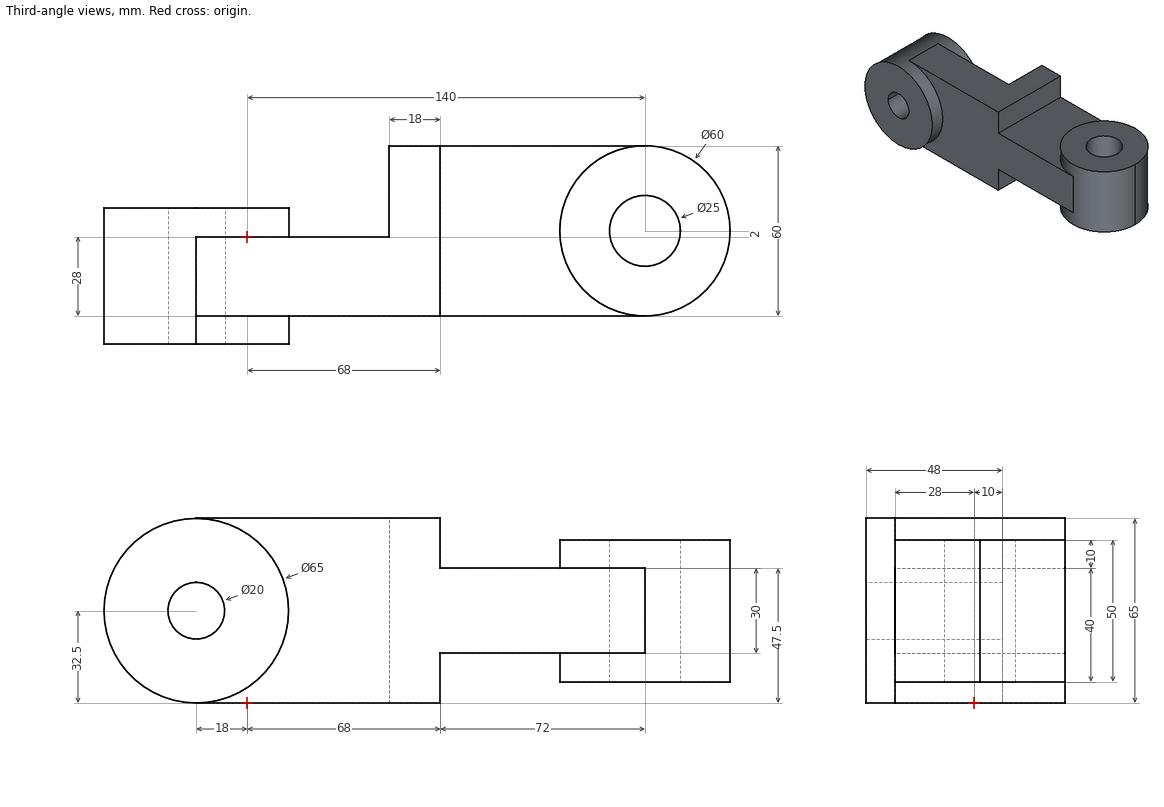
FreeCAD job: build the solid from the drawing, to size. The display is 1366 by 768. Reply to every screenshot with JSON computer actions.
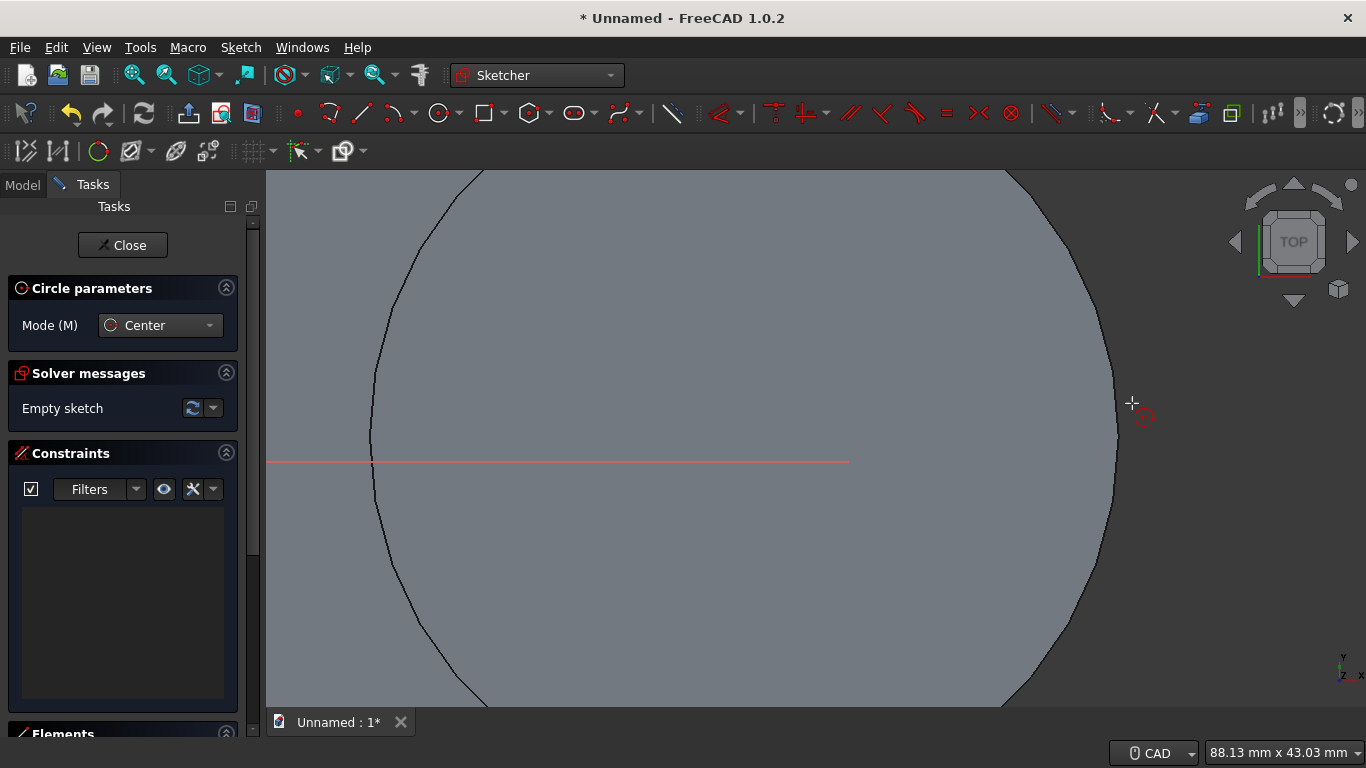
{"action": "left_click", "coordinate": [744, 437]}
{"action": "left_click", "coordinate": [855, 326]}
{"action": "key", "text": "Escape"}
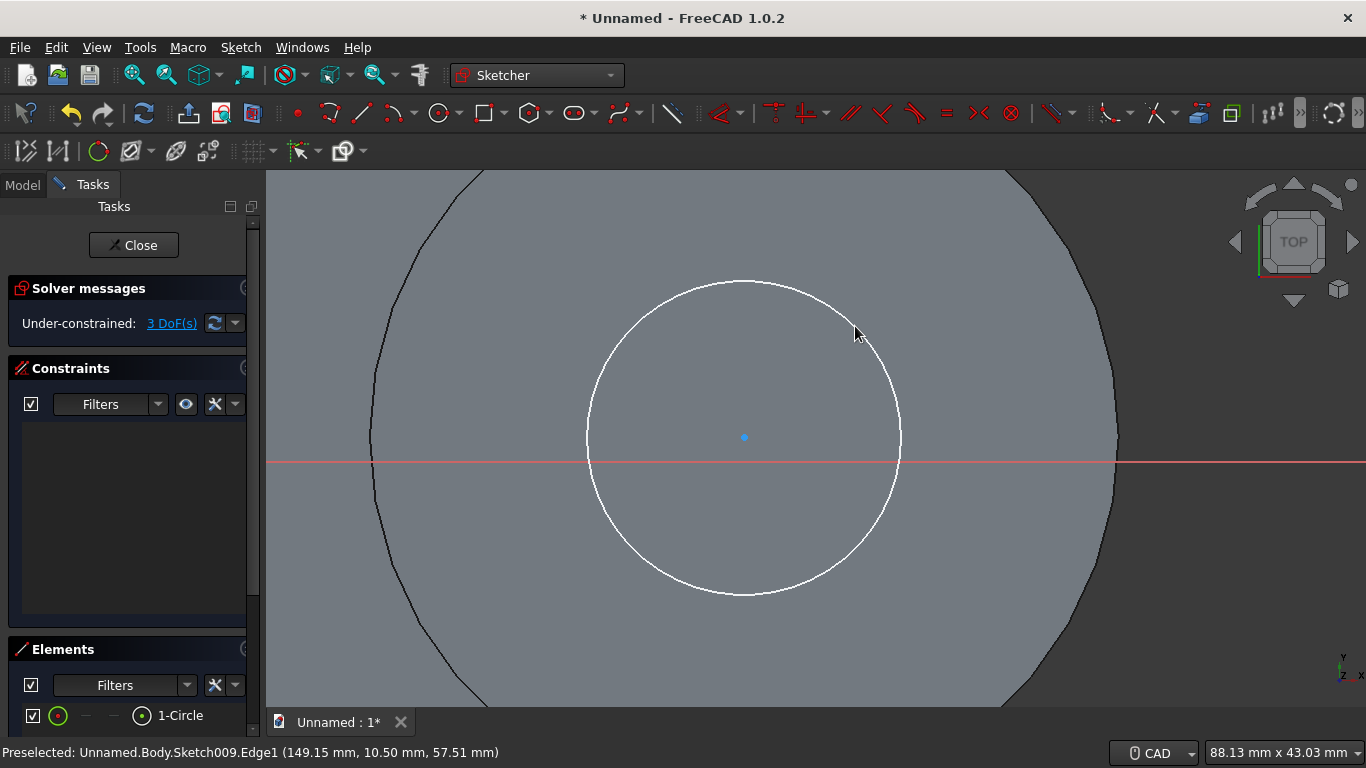
{"action": "key", "text": "d"}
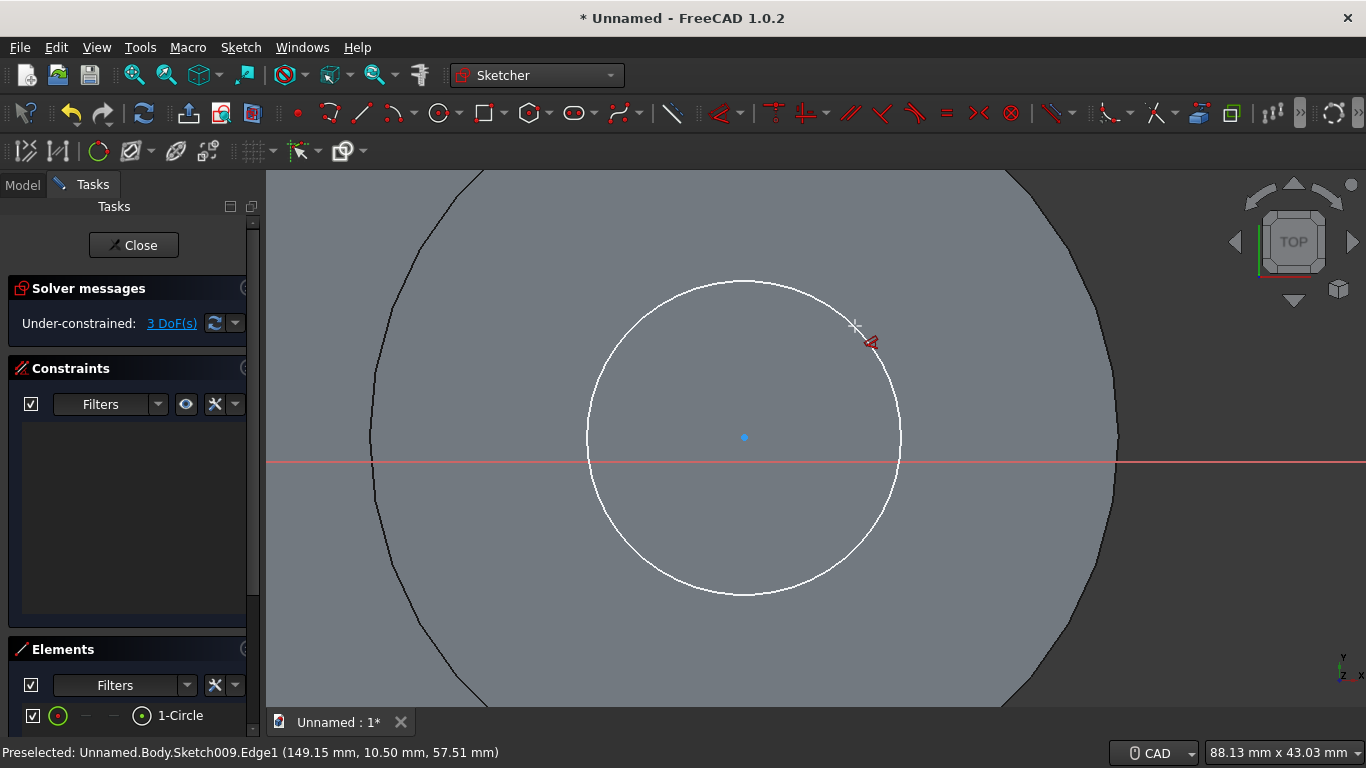
{"action": "left_click", "coordinate": [855, 327]}
{"action": "left_click", "coordinate": [878, 304]}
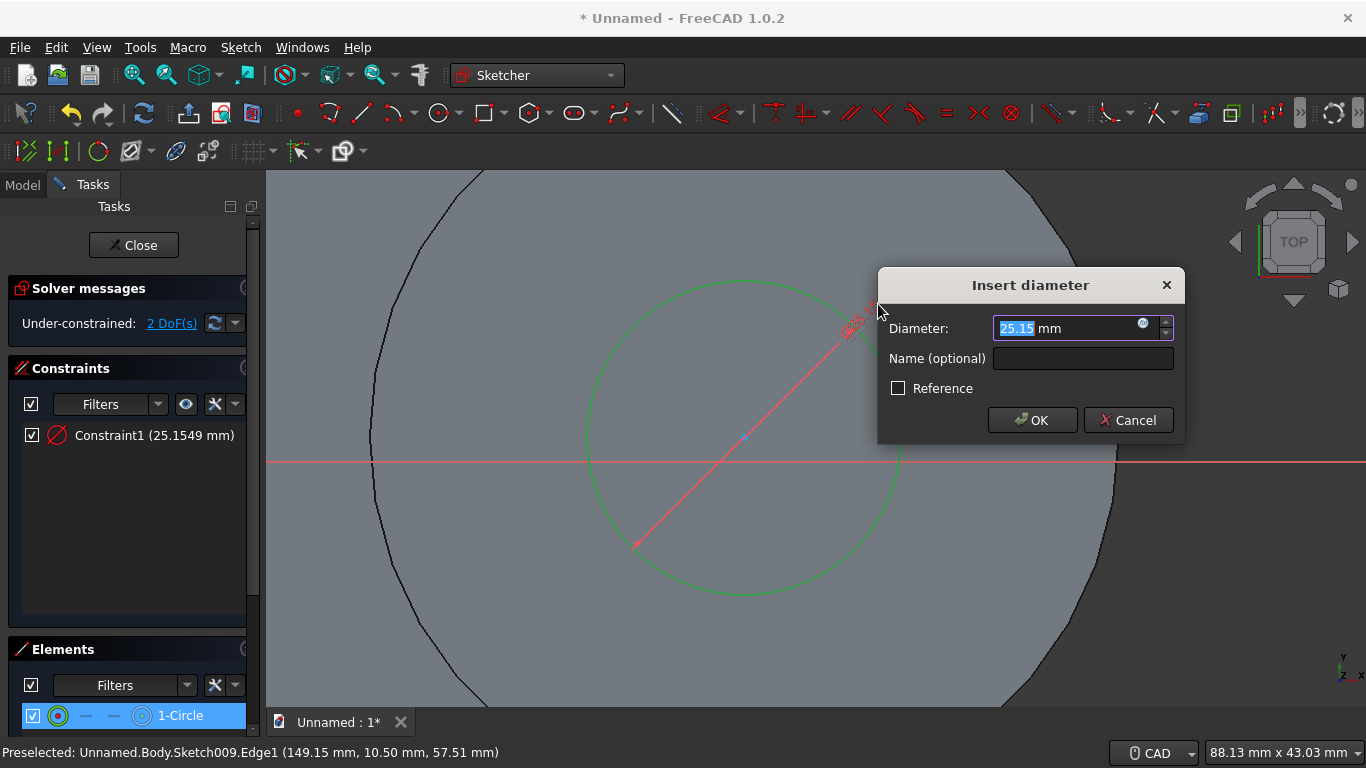
{"action": "type", "text": "25"}
{"action": "key", "text": "Return"}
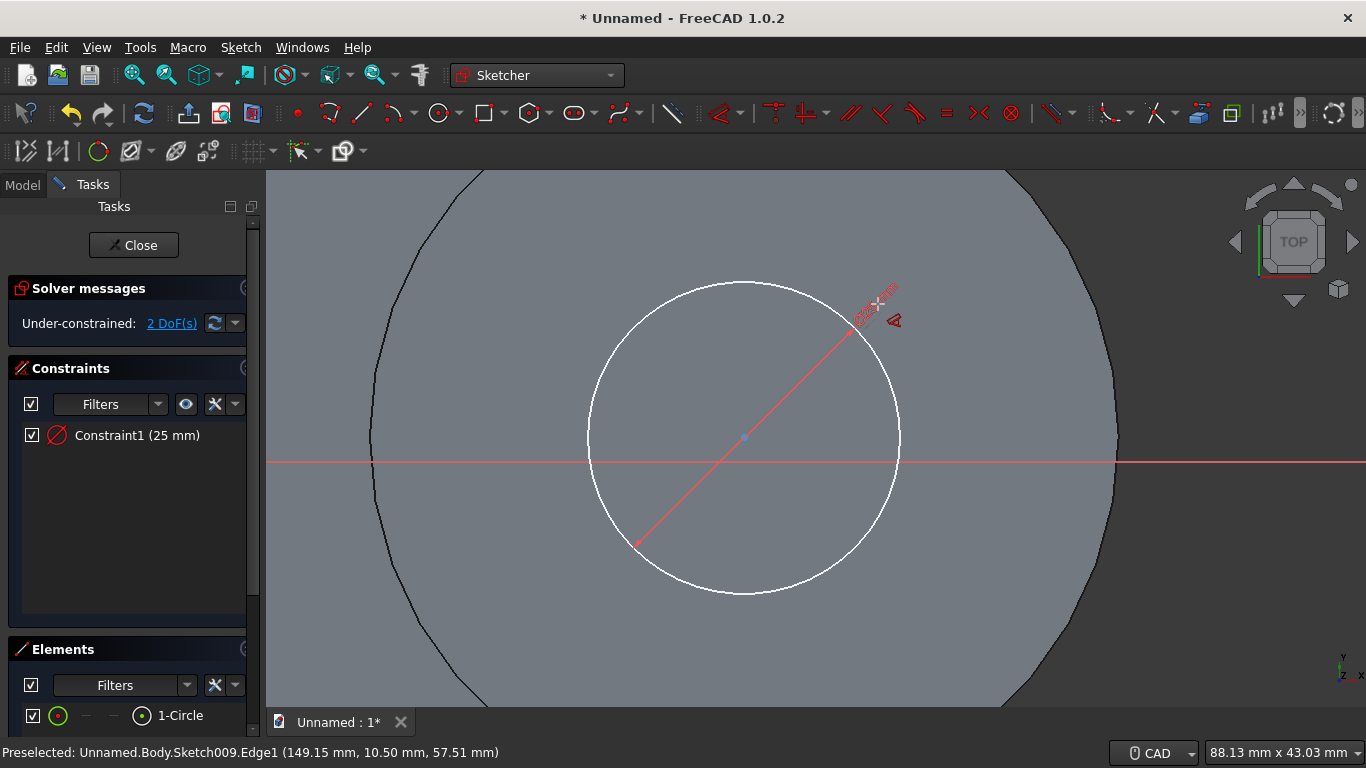
{"action": "scroll", "coordinate": [744, 438], "scroll_direction": "up", "scroll_amount": 3}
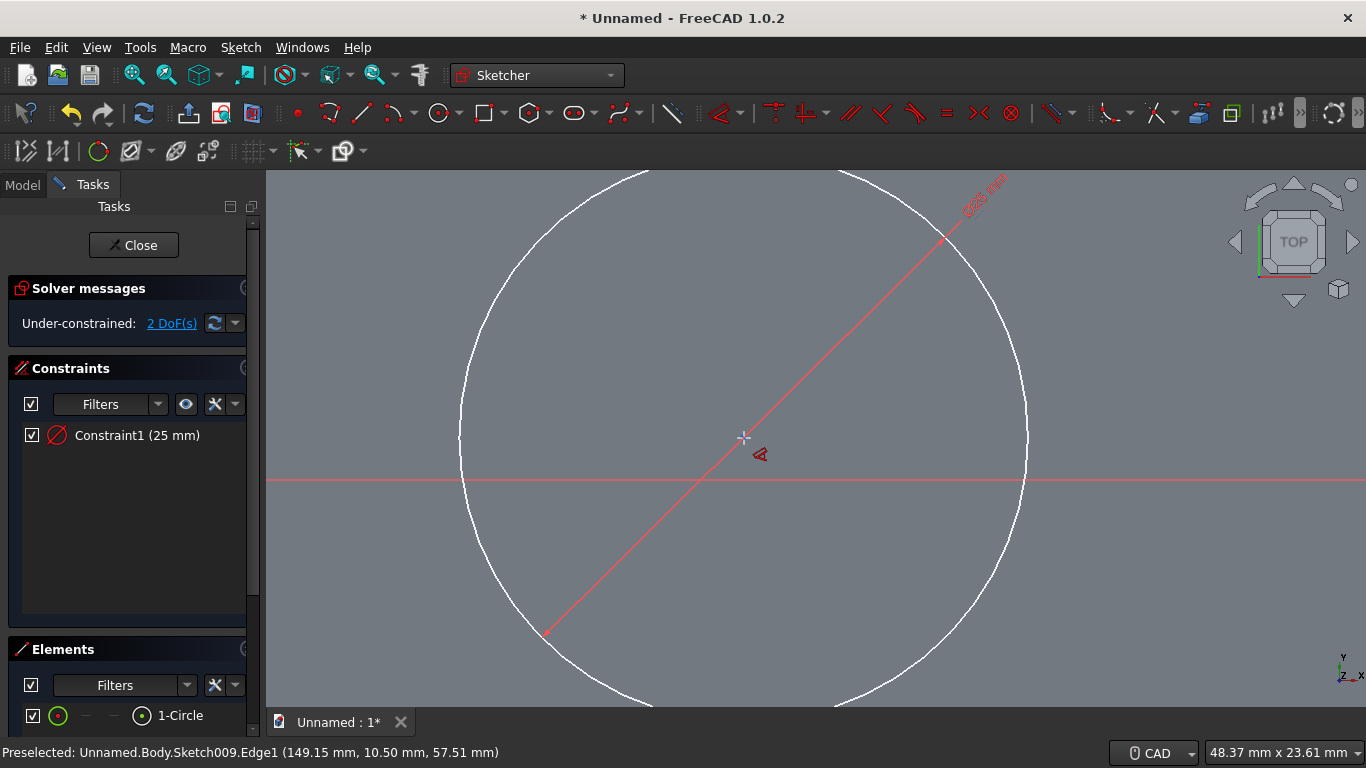
{"action": "left_click", "coordinate": [744, 438]}
{"action": "left_click", "coordinate": [778, 459]}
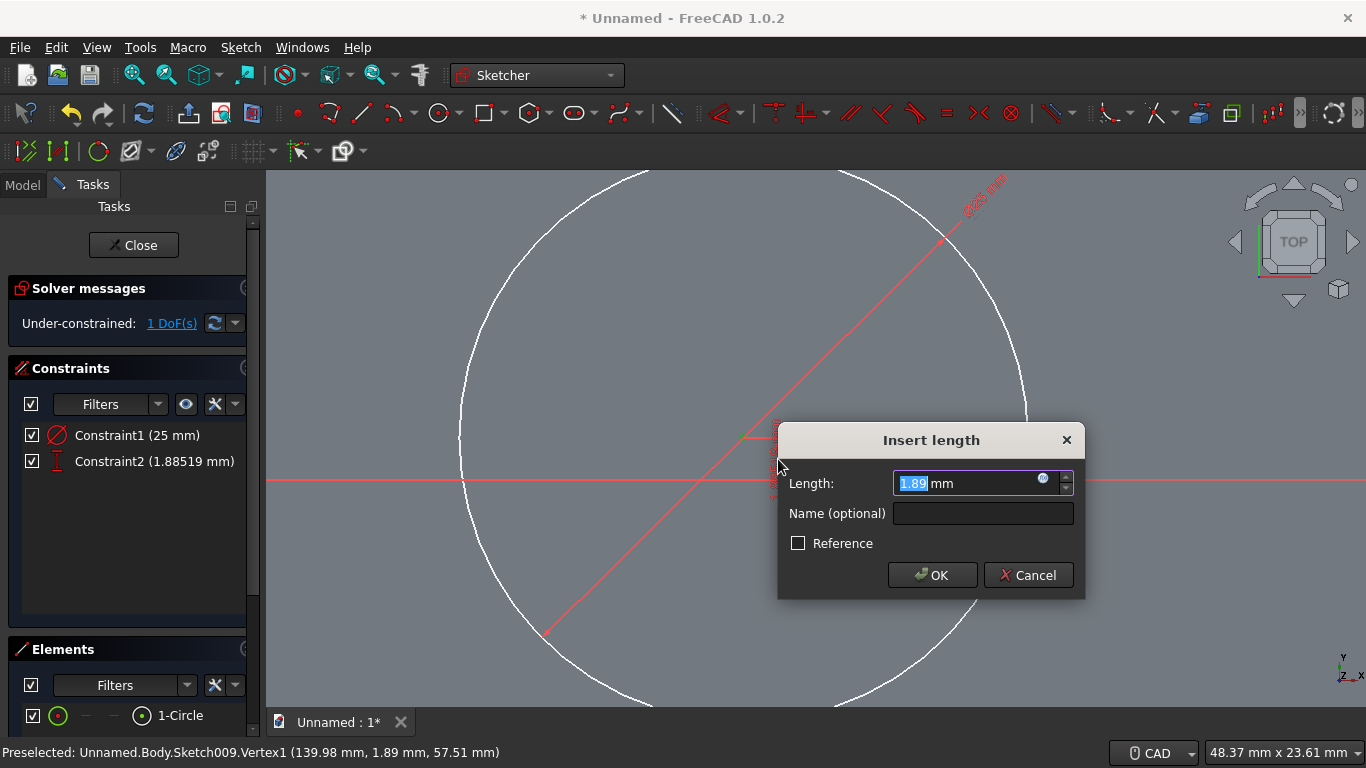
{"action": "type", "text": "2"}
{"action": "key", "text": "Return"}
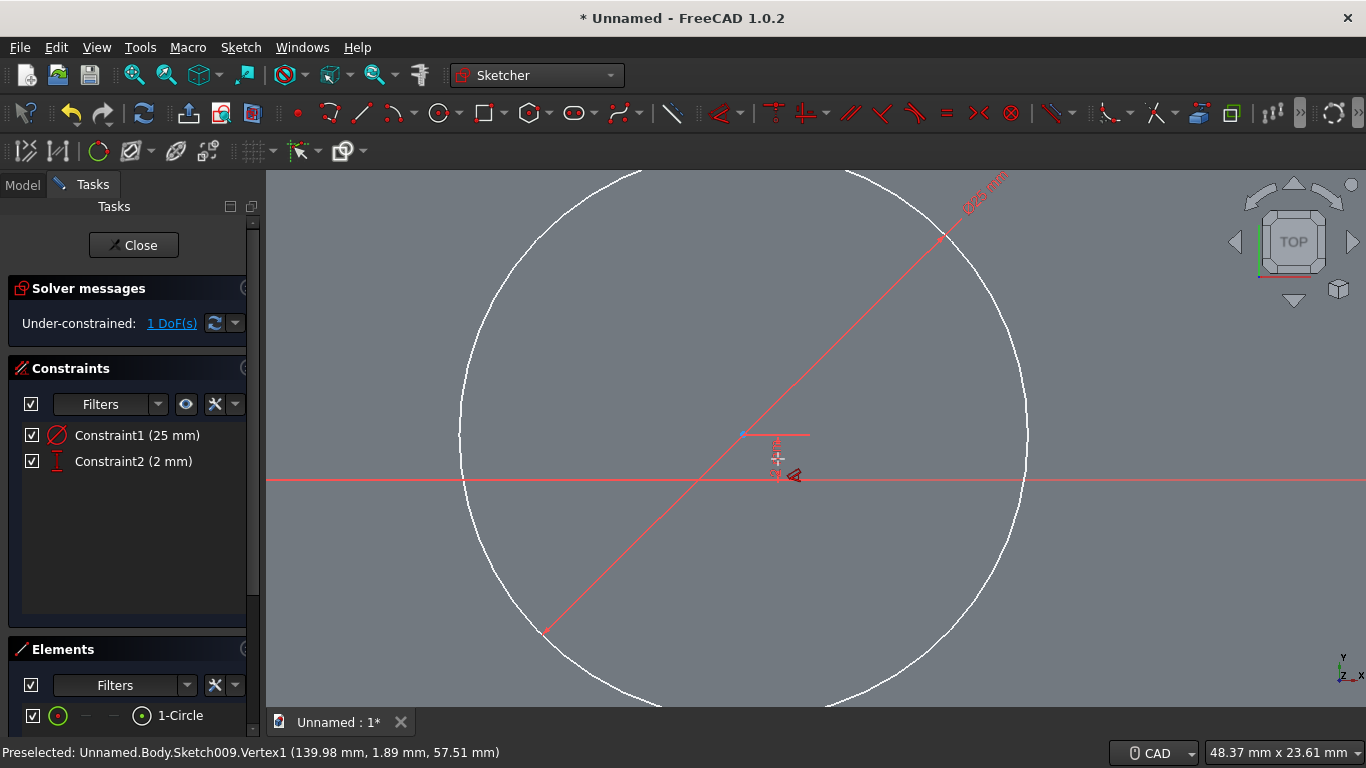
{"action": "left_click", "coordinate": [744, 435]}
{"action": "left_click", "coordinate": [519, 514]}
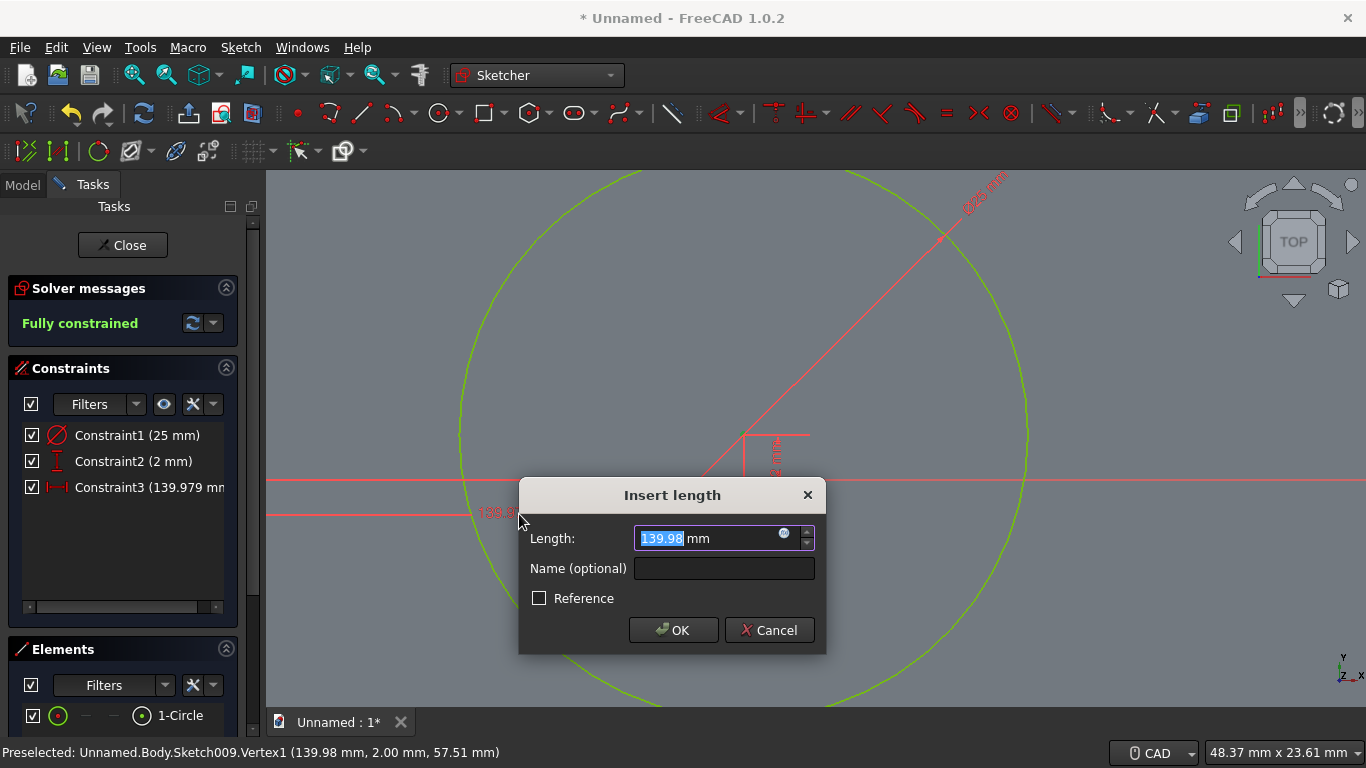
{"action": "type", "text": "140"}
{"action": "key", "text": "Return"}
{"action": "key", "text": "Escape"}